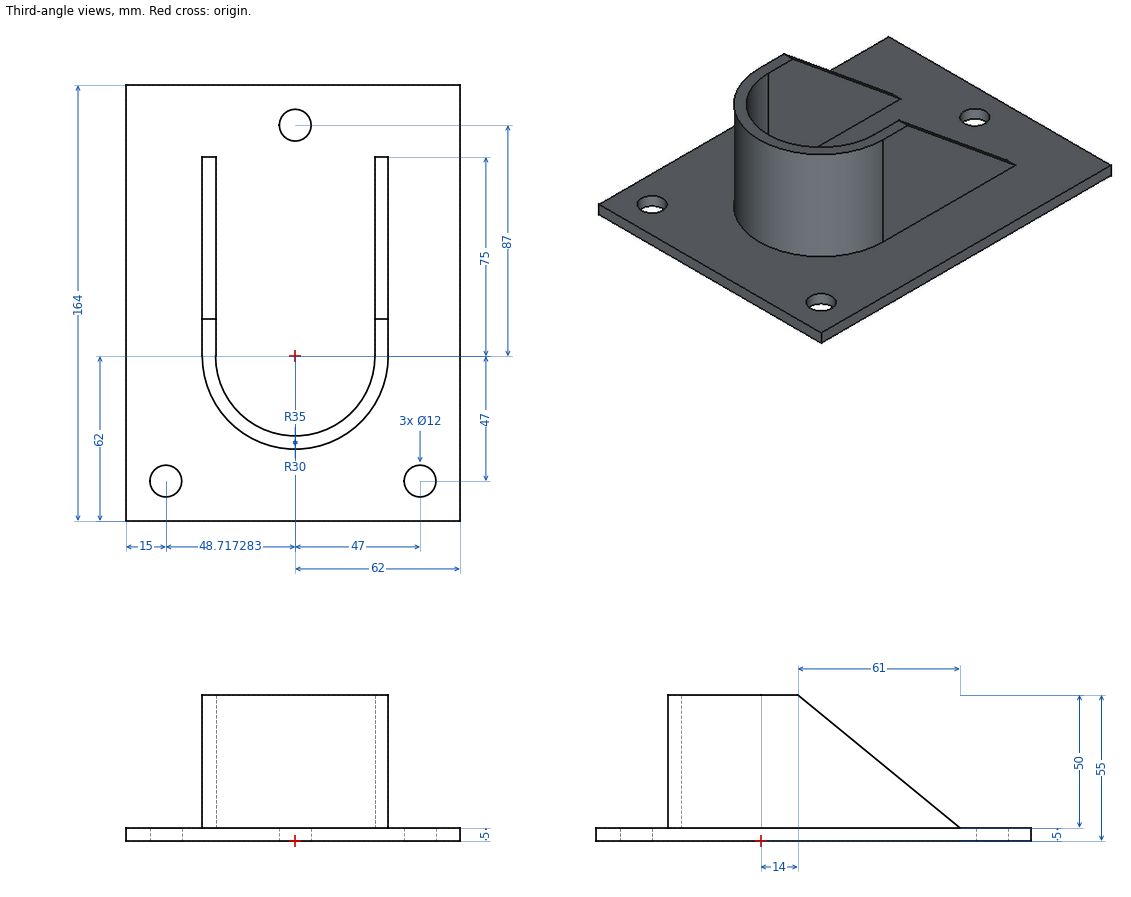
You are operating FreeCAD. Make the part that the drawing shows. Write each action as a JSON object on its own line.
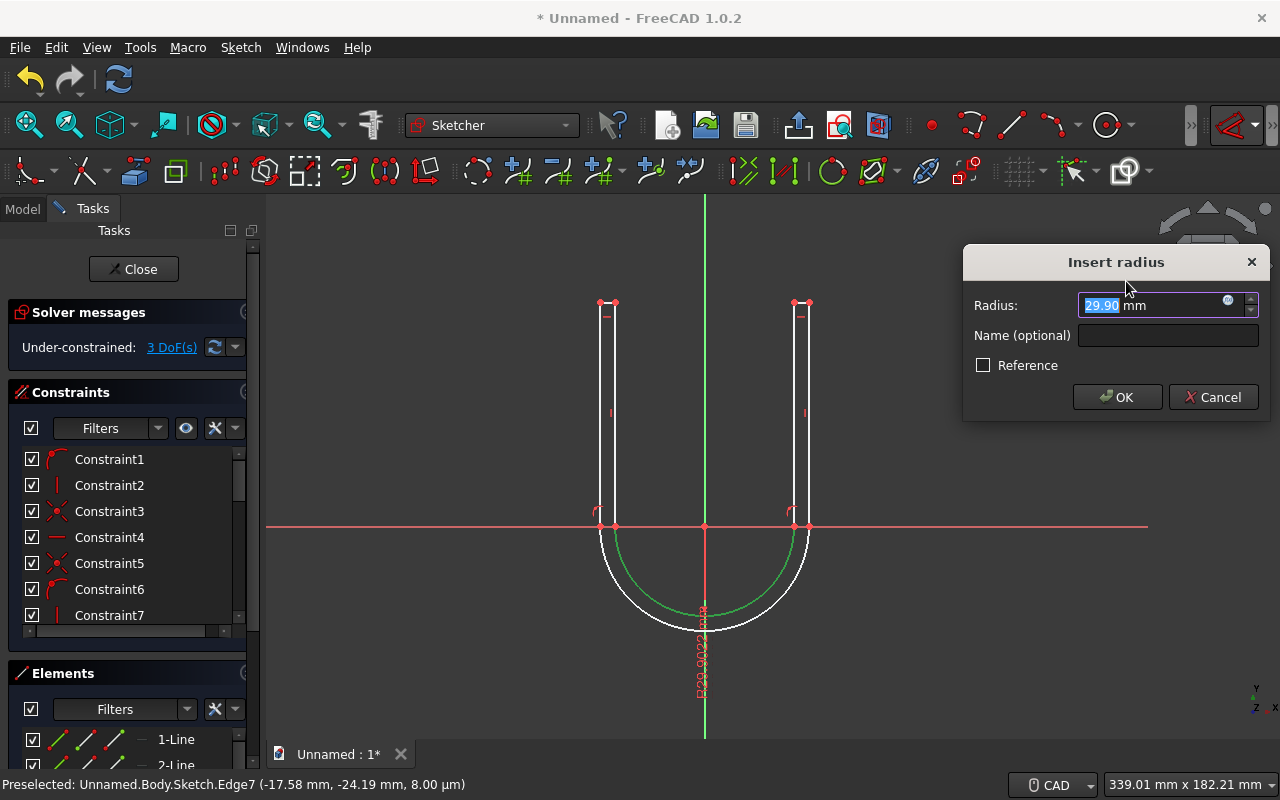
{"action": "type", "text": "30"}
{"action": "key", "text": "Return"}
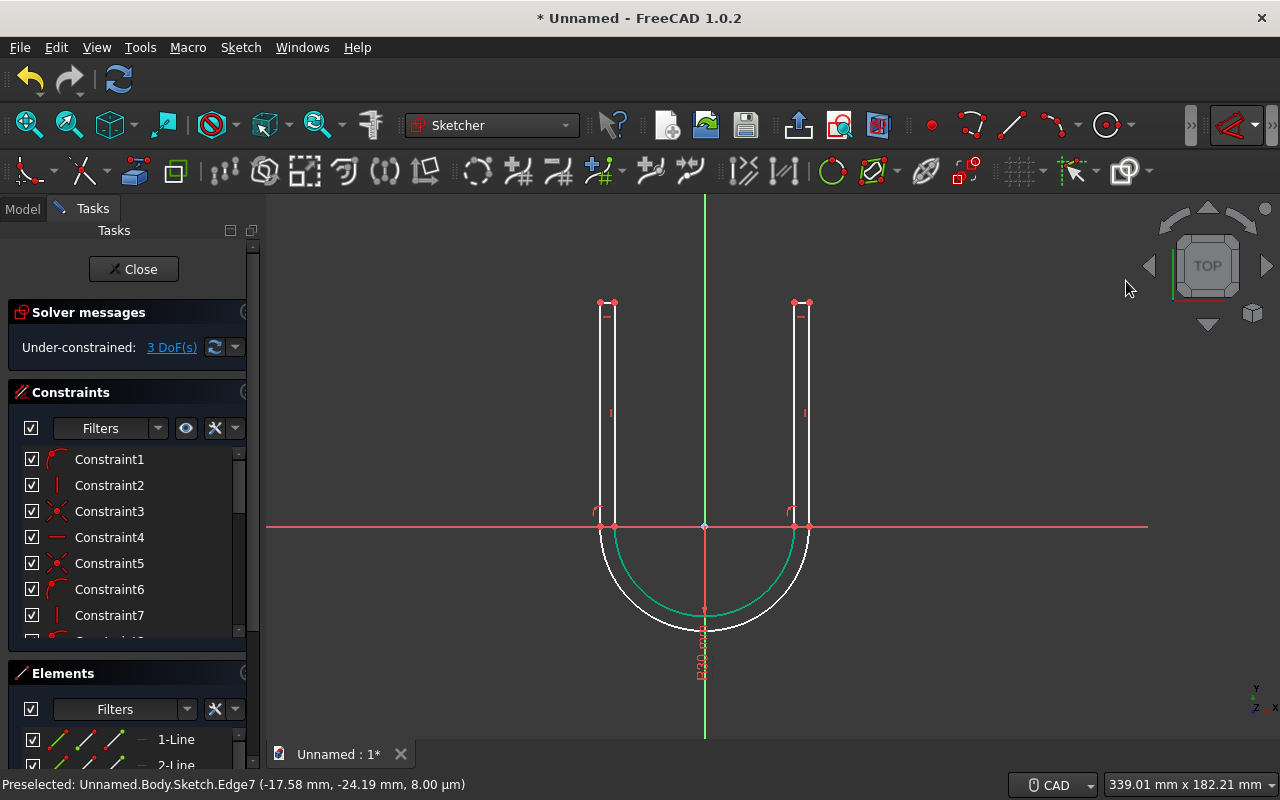
{"action": "left_click", "coordinate": [643, 611]}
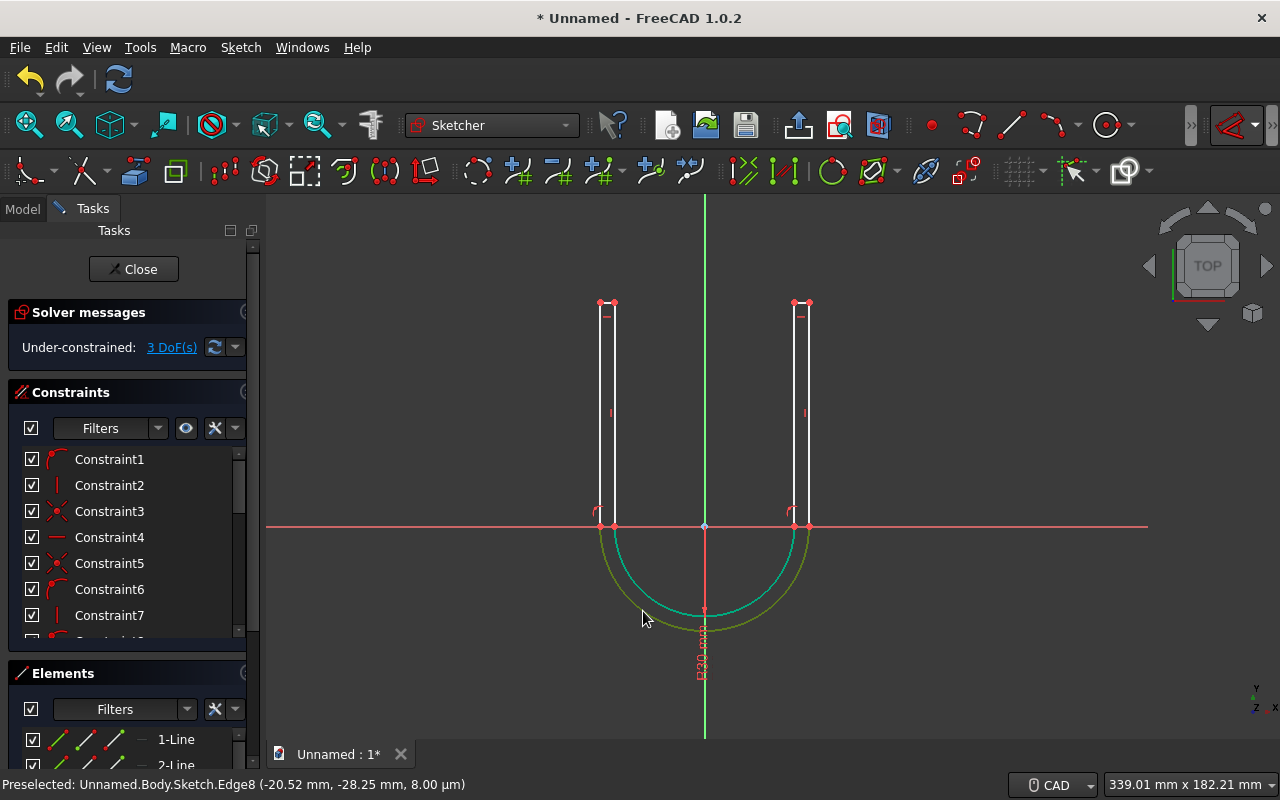
{"action": "left_click", "coordinate": [1258, 126]}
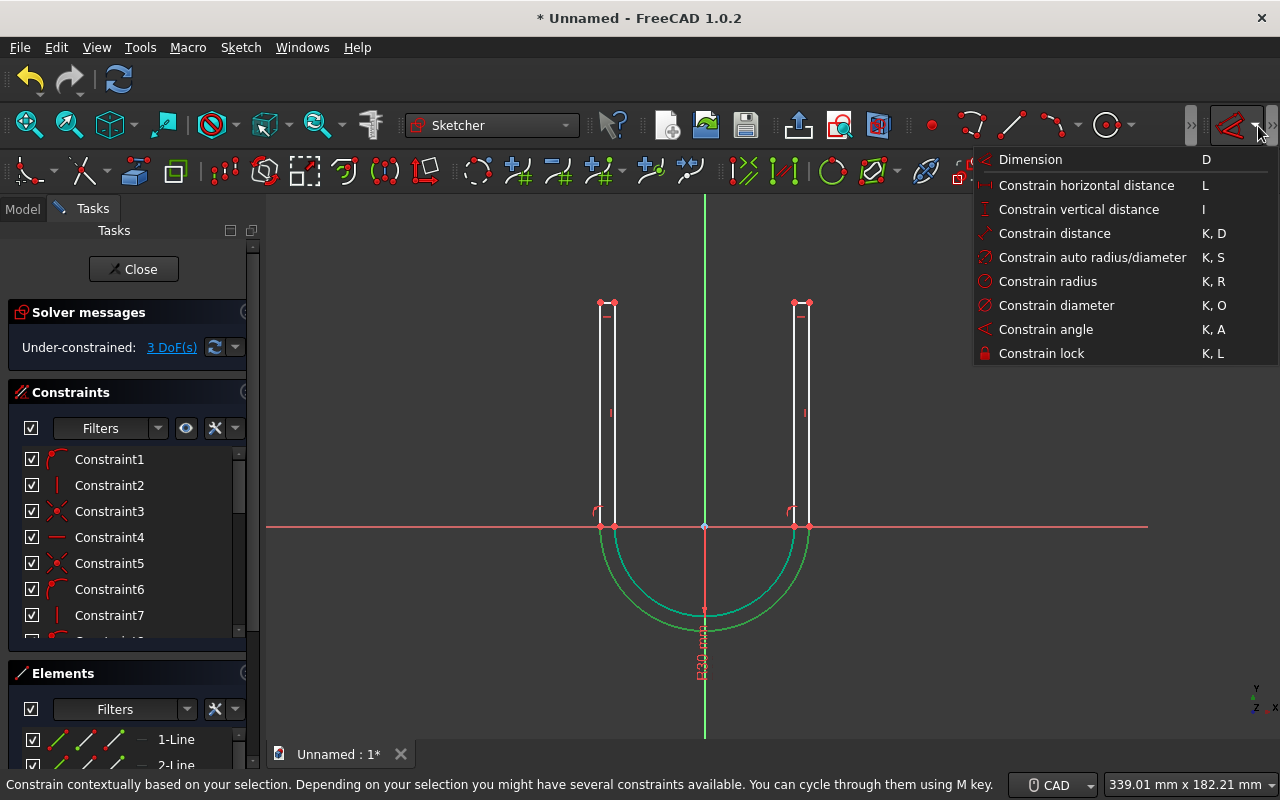
{"action": "left_click", "coordinate": [1126, 281]}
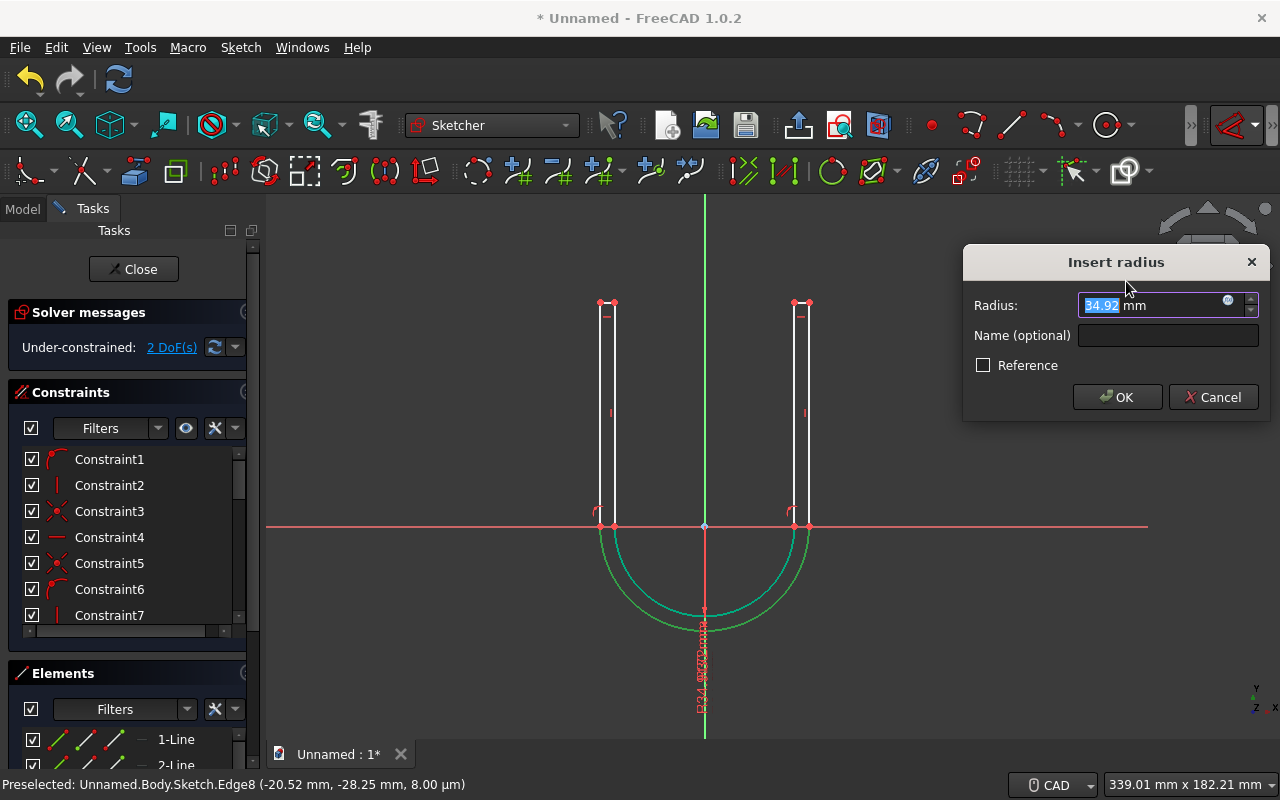
{"action": "type", "text": "35"}
{"action": "key", "text": "Return"}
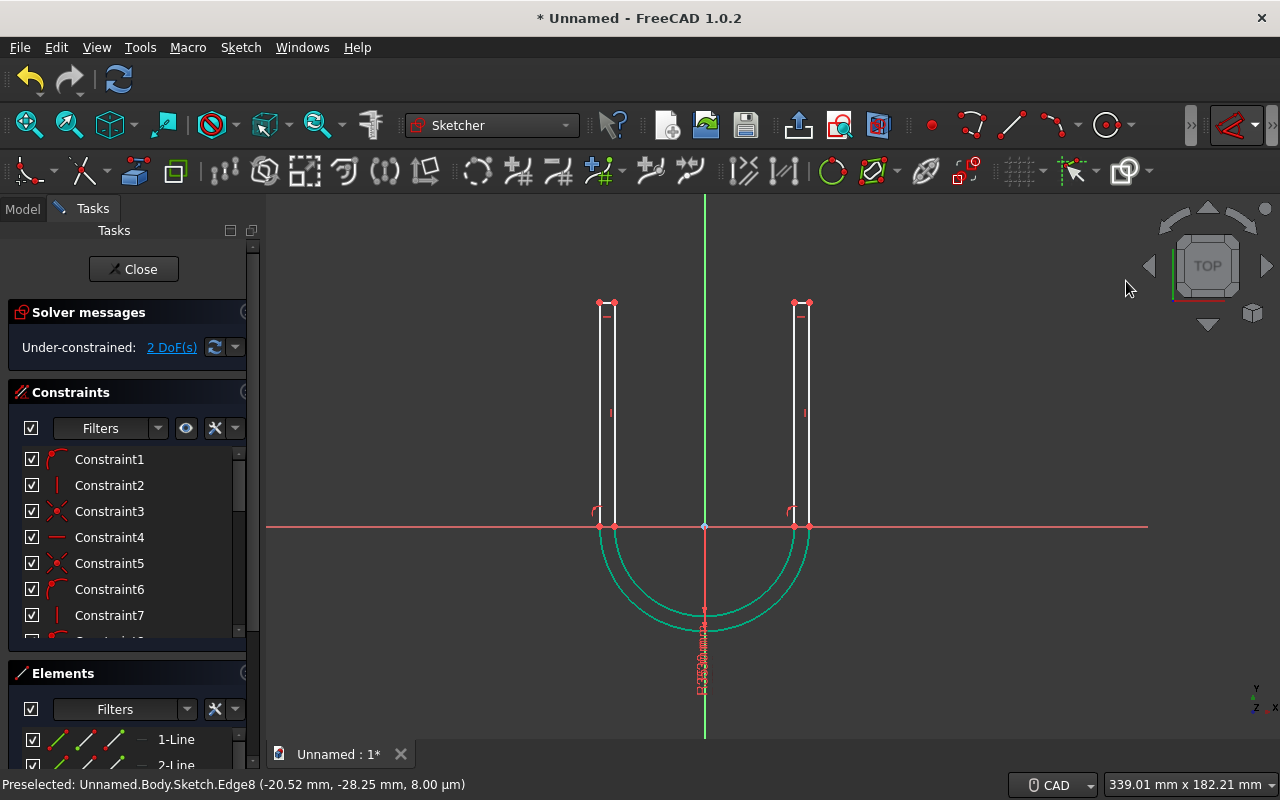
{"action": "left_click", "coordinate": [809, 460]}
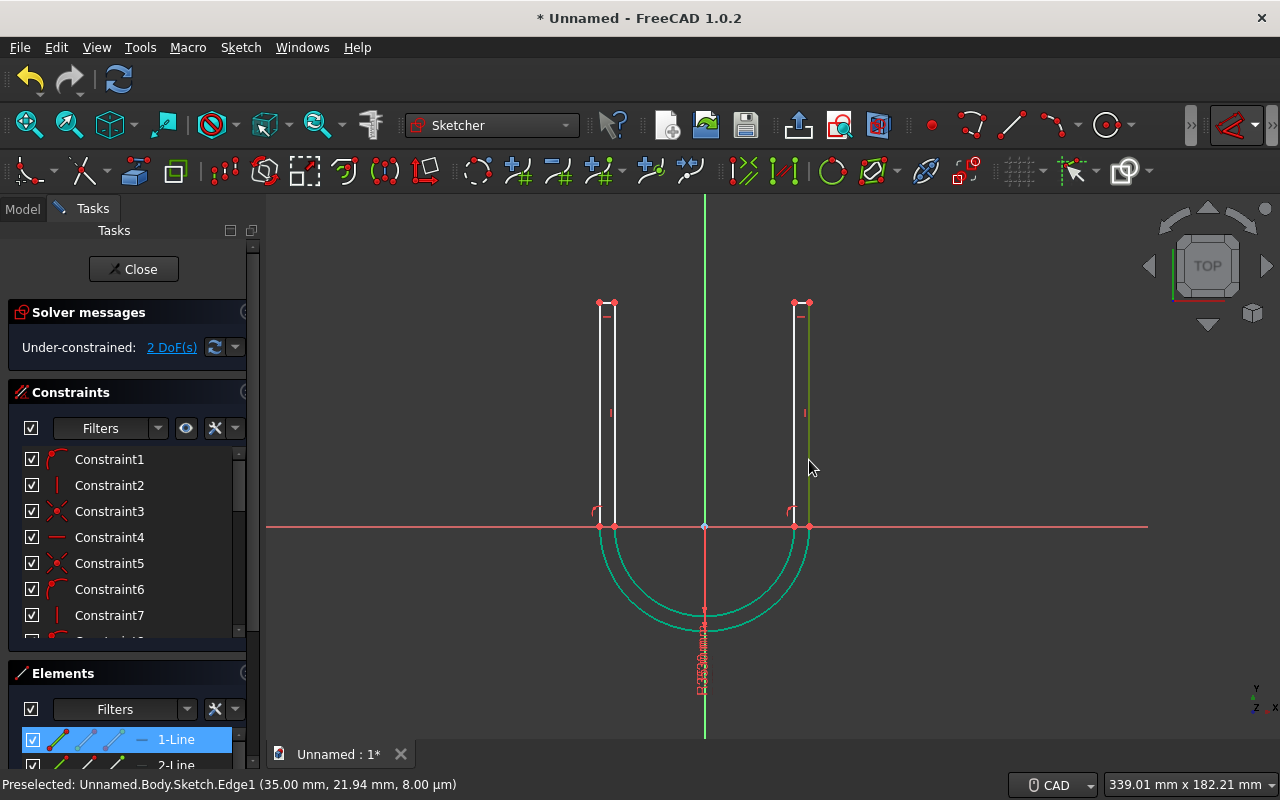
{"action": "key", "text": "i"}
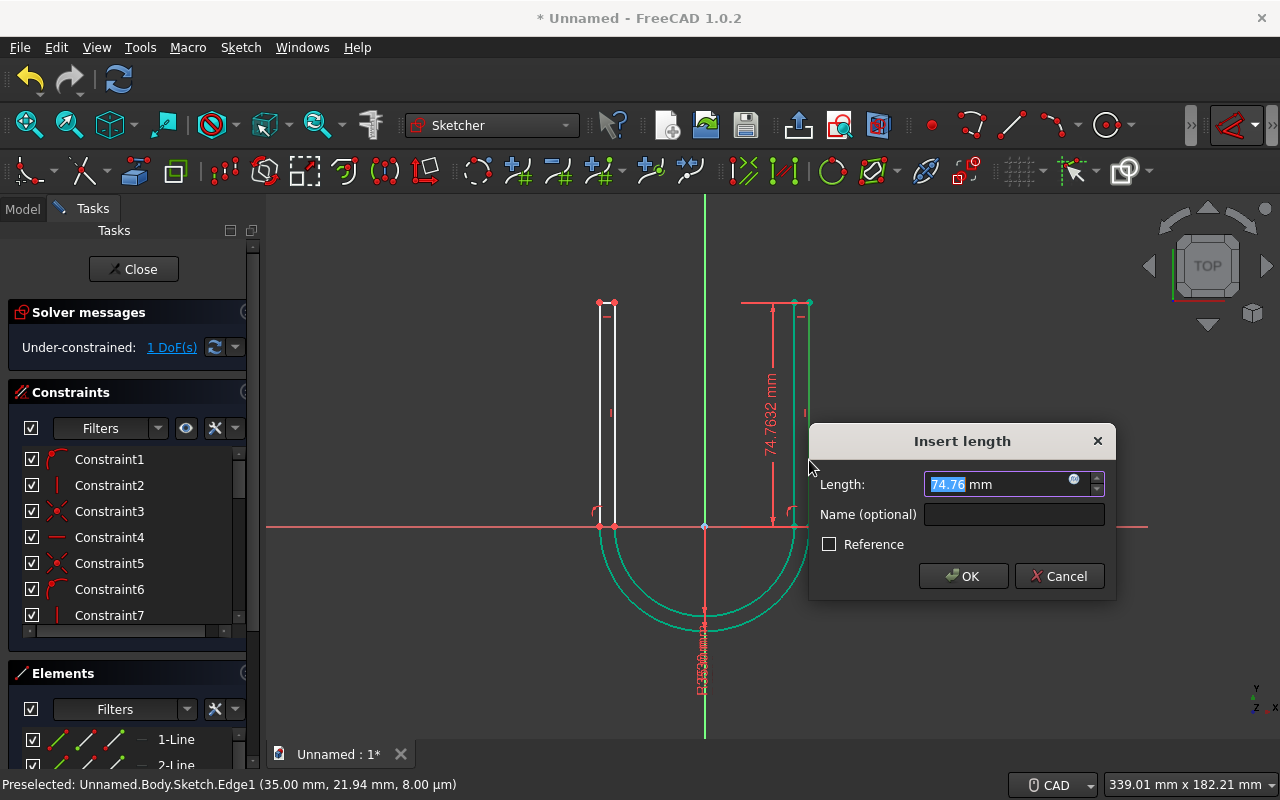
{"action": "type", "text": "75"}
{"action": "key", "text": "Return"}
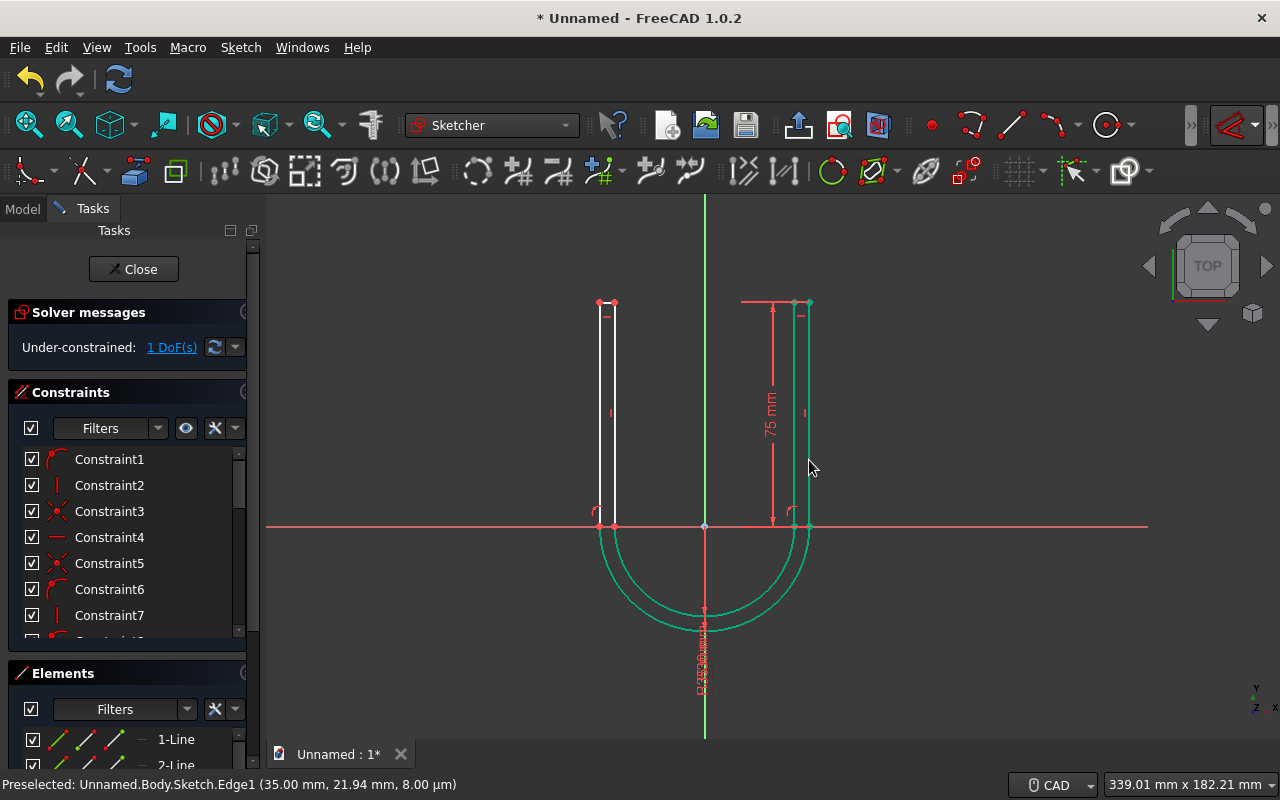
{"action": "left_click", "coordinate": [615, 460]}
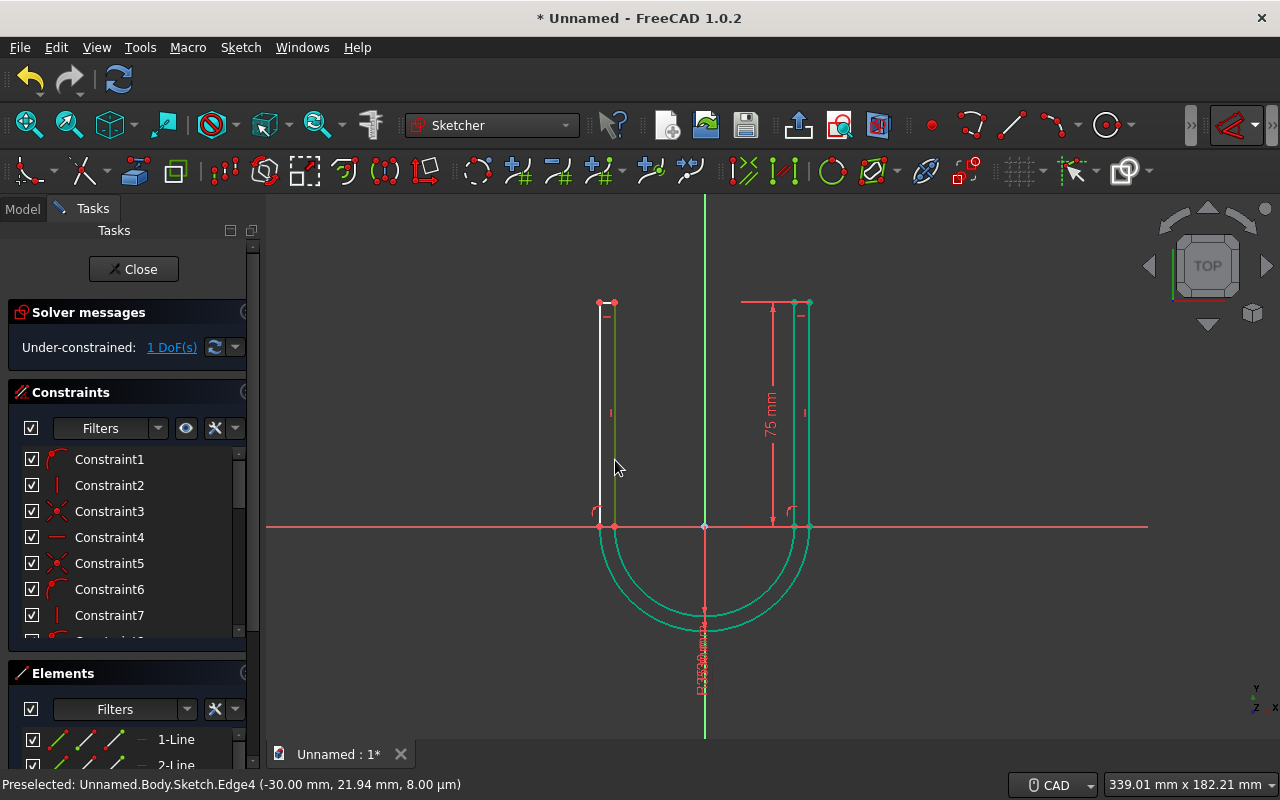
{"action": "left_click", "coordinate": [1258, 126]}